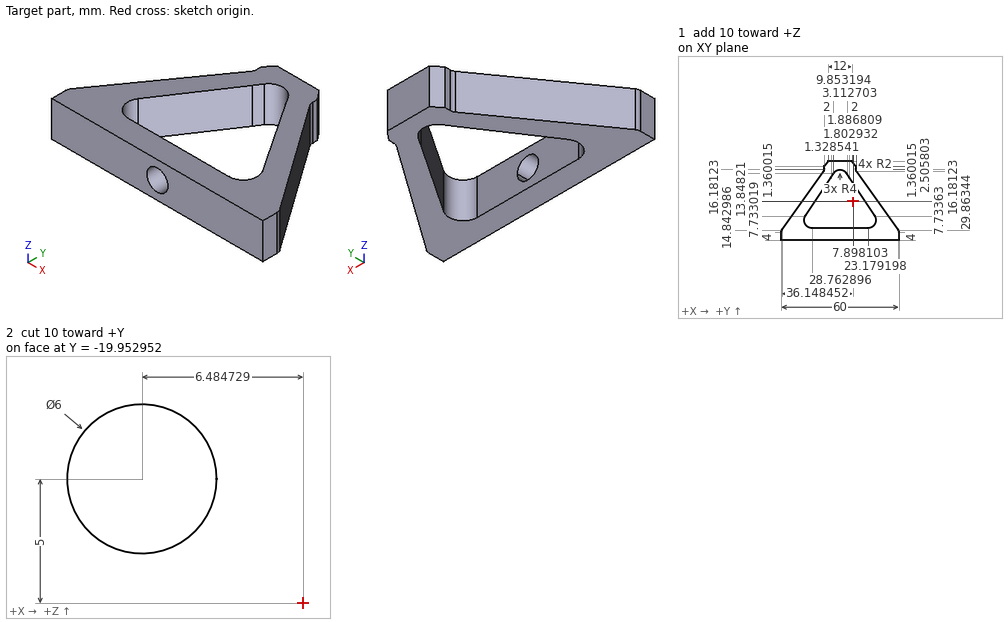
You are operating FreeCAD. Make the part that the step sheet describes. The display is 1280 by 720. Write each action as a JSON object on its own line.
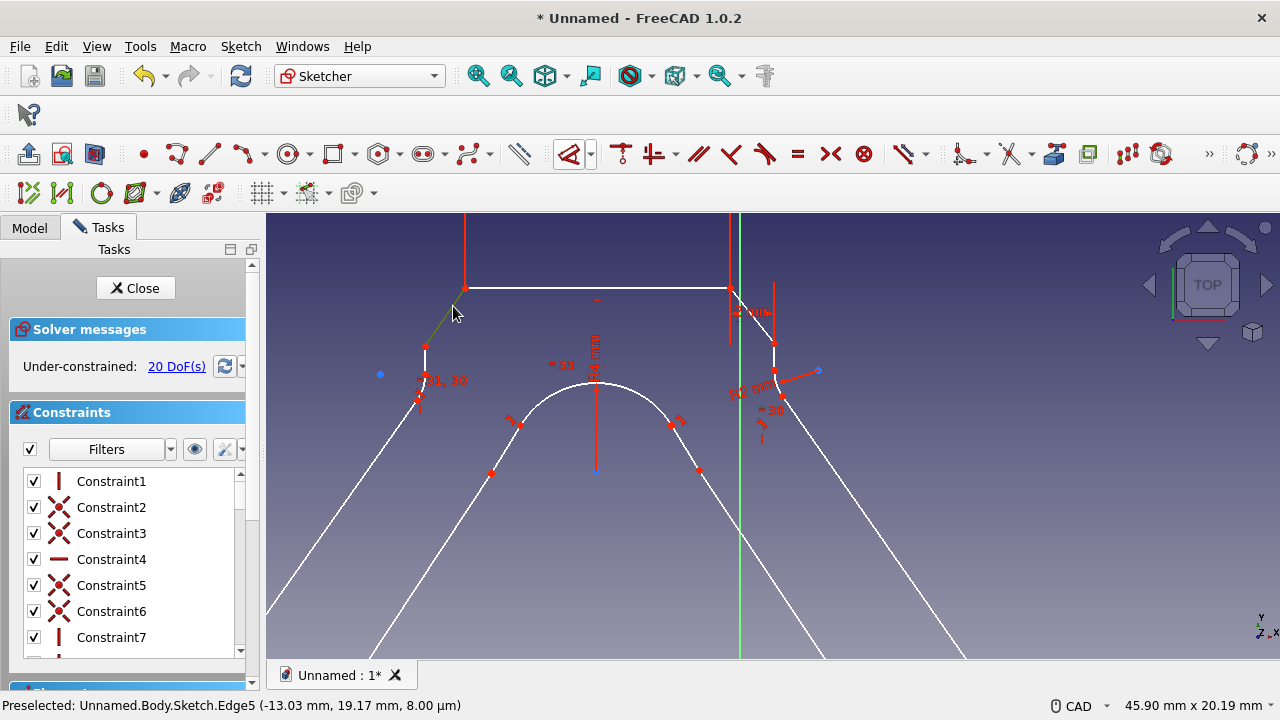
{"action": "key", "text": "l"}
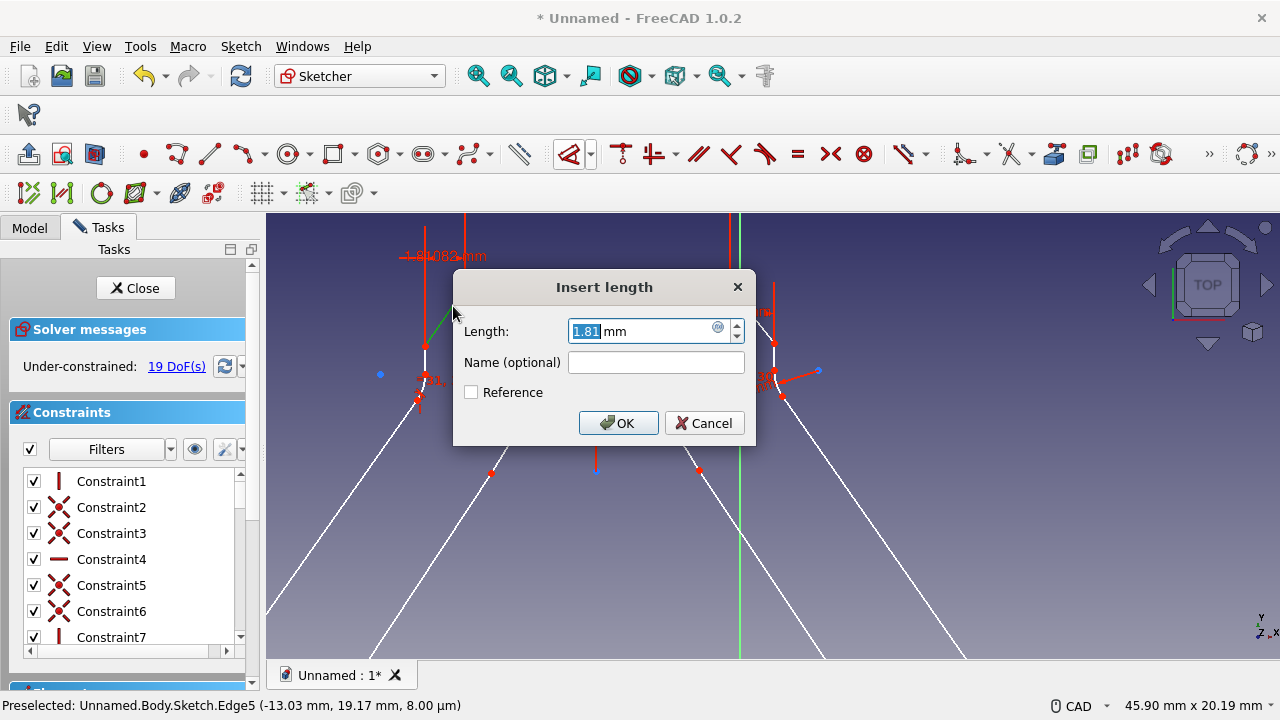
{"action": "type", "text": "2"}
{"action": "key", "text": "Return"}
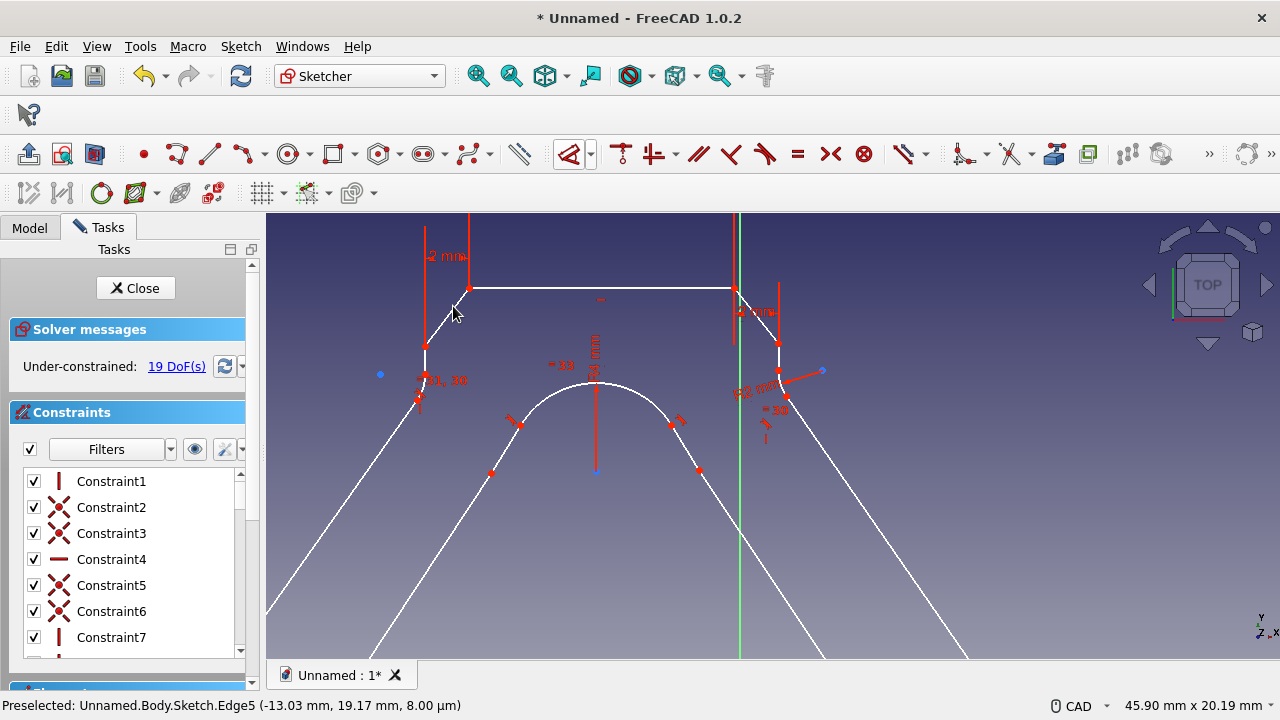
{"action": "scroll", "coordinate": [779, 360], "scroll_direction": "up", "scroll_amount": 2}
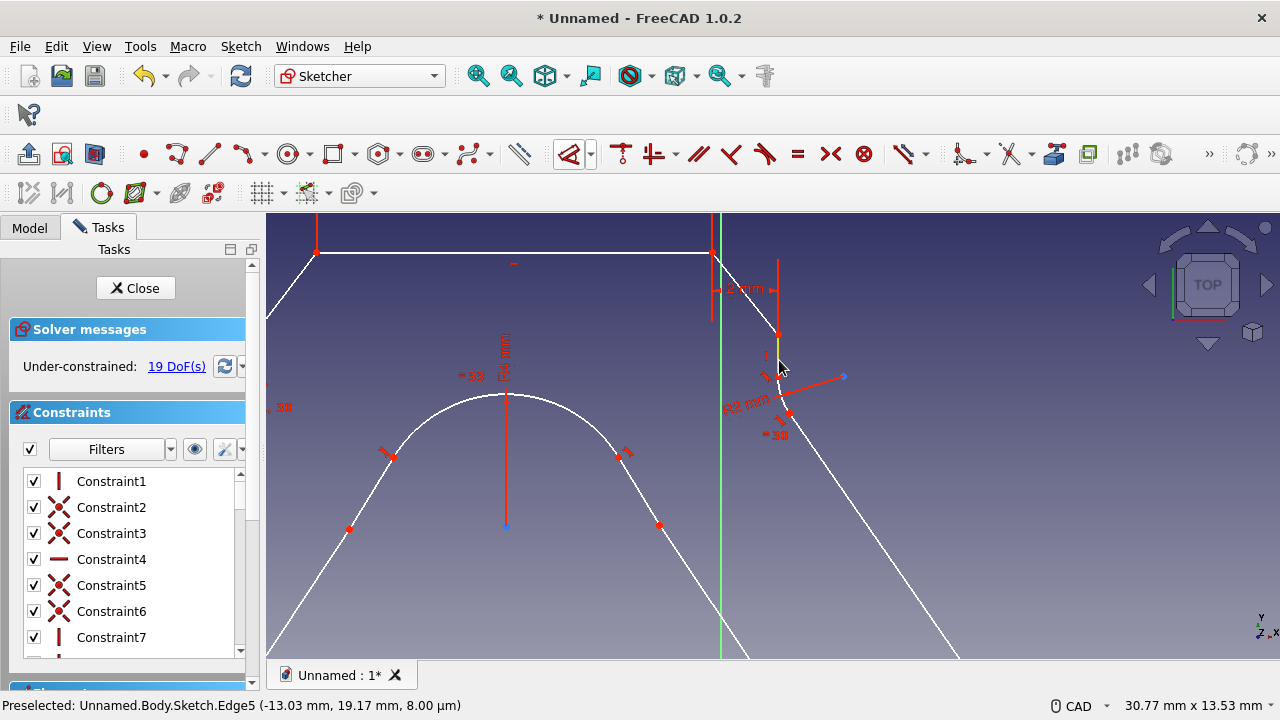
{"action": "left_click", "coordinate": [778, 360]}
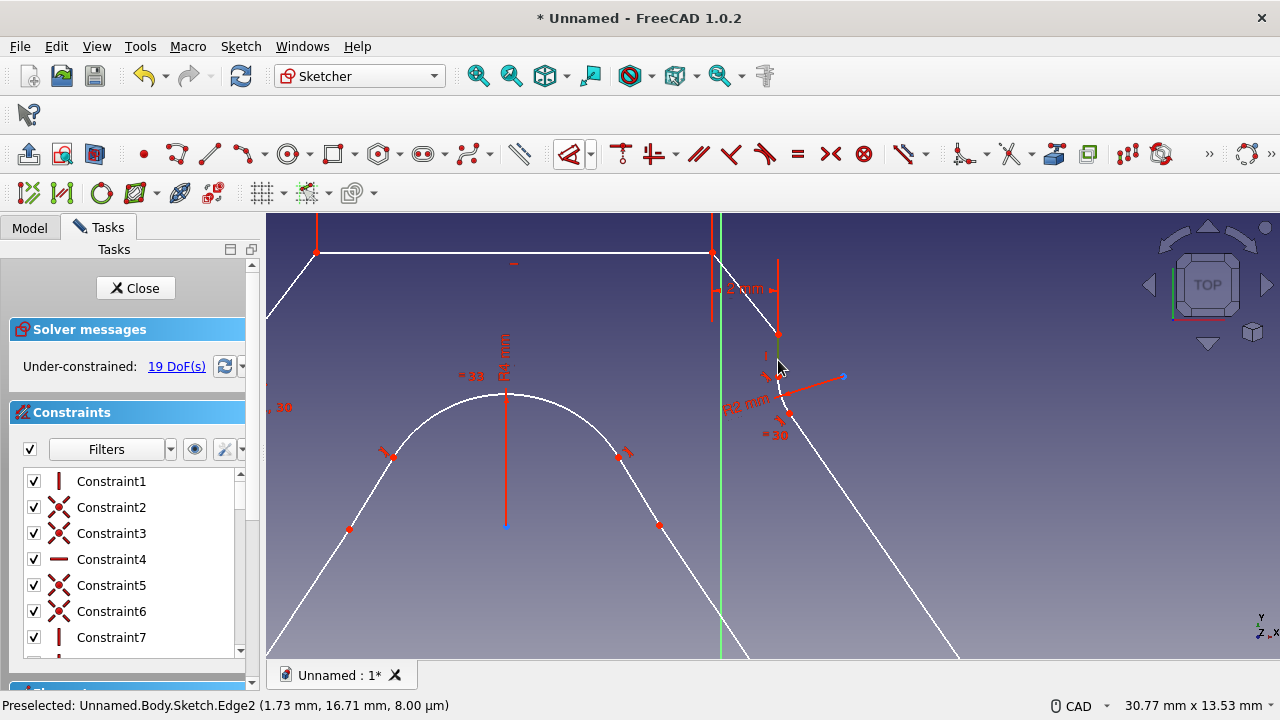
{"action": "key", "text": "i"}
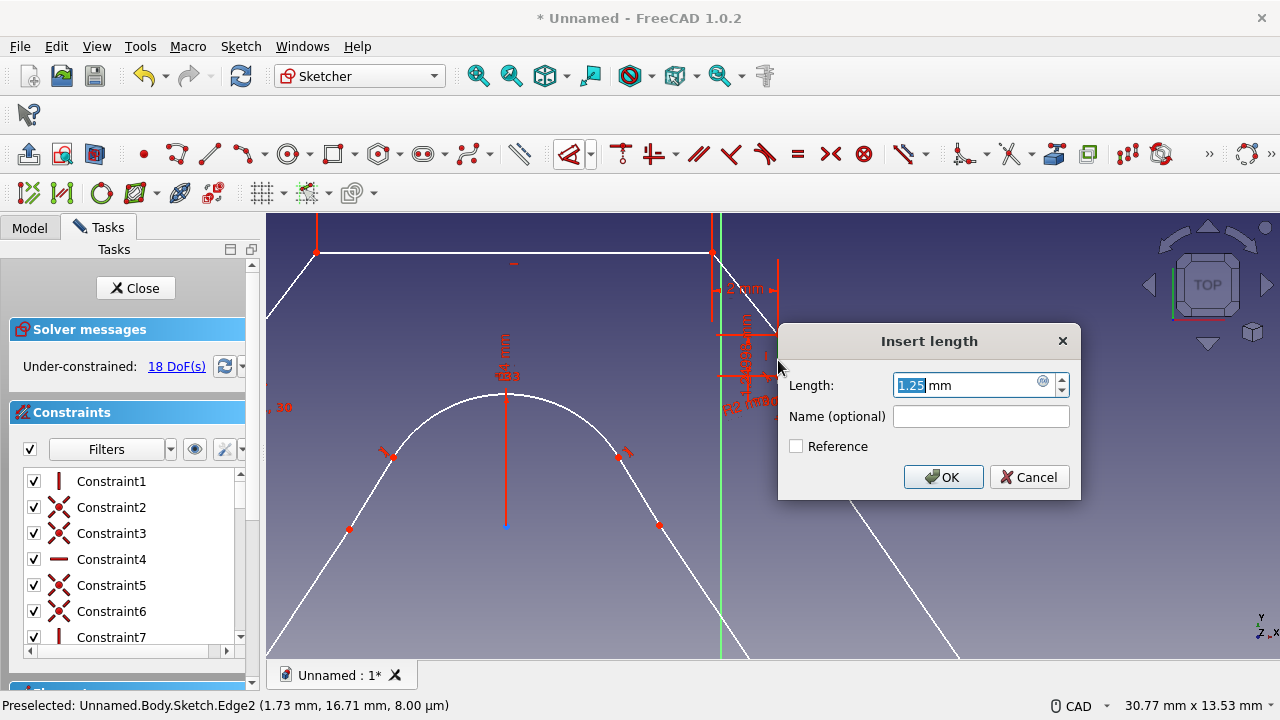
{"action": "type", "text": "1.360015"}
{"action": "key", "text": "Return"}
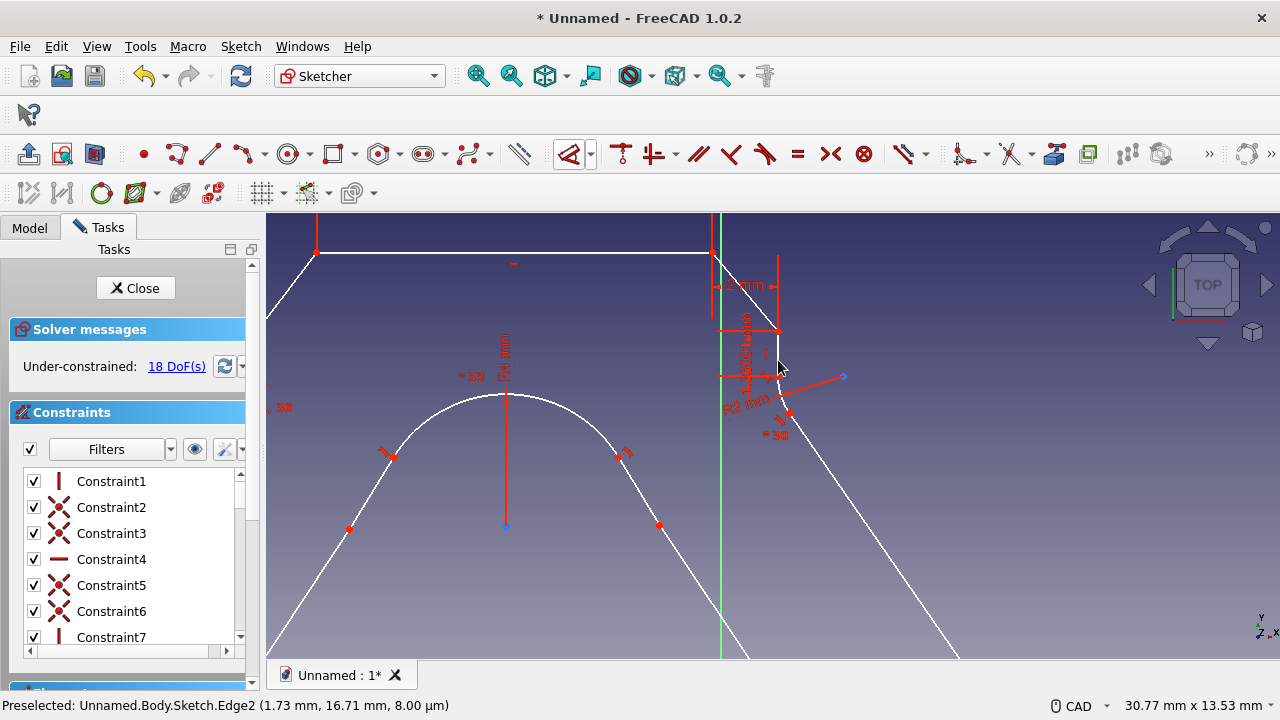
{"action": "scroll", "coordinate": [754, 316], "scroll_direction": "down", "scroll_amount": 8}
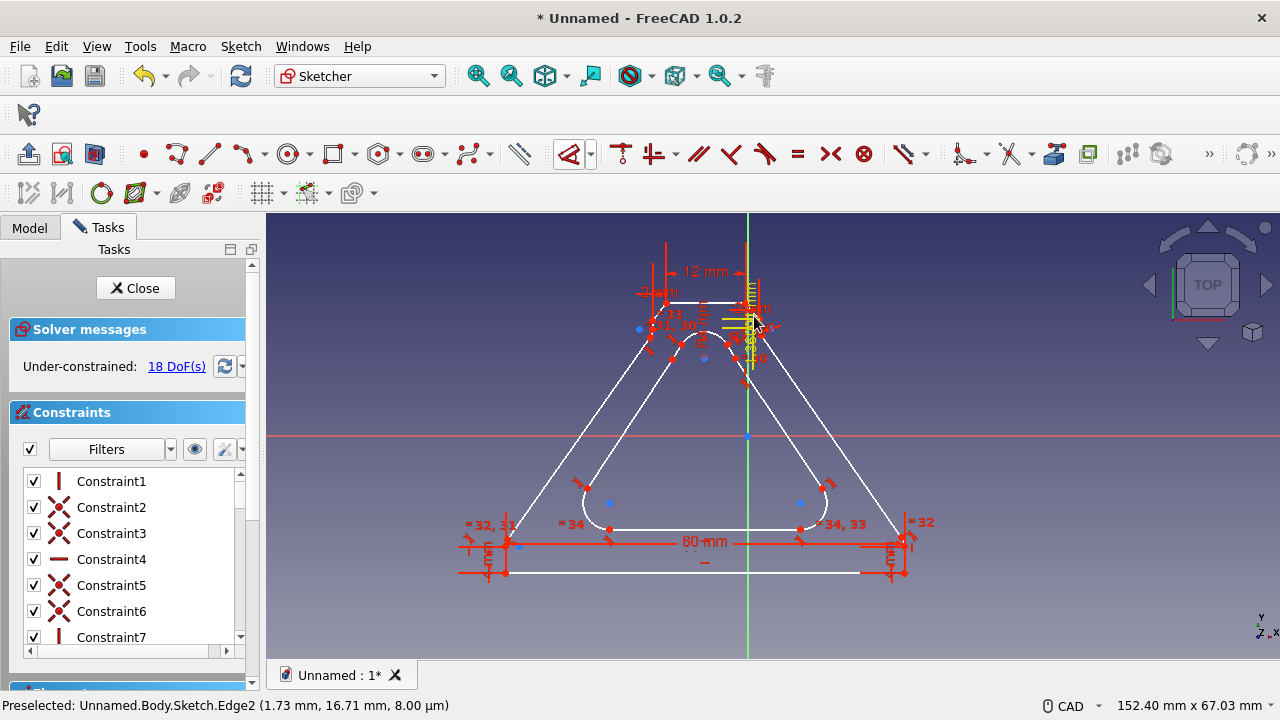
{"action": "scroll", "coordinate": [653, 323], "scroll_direction": "up", "scroll_amount": 9}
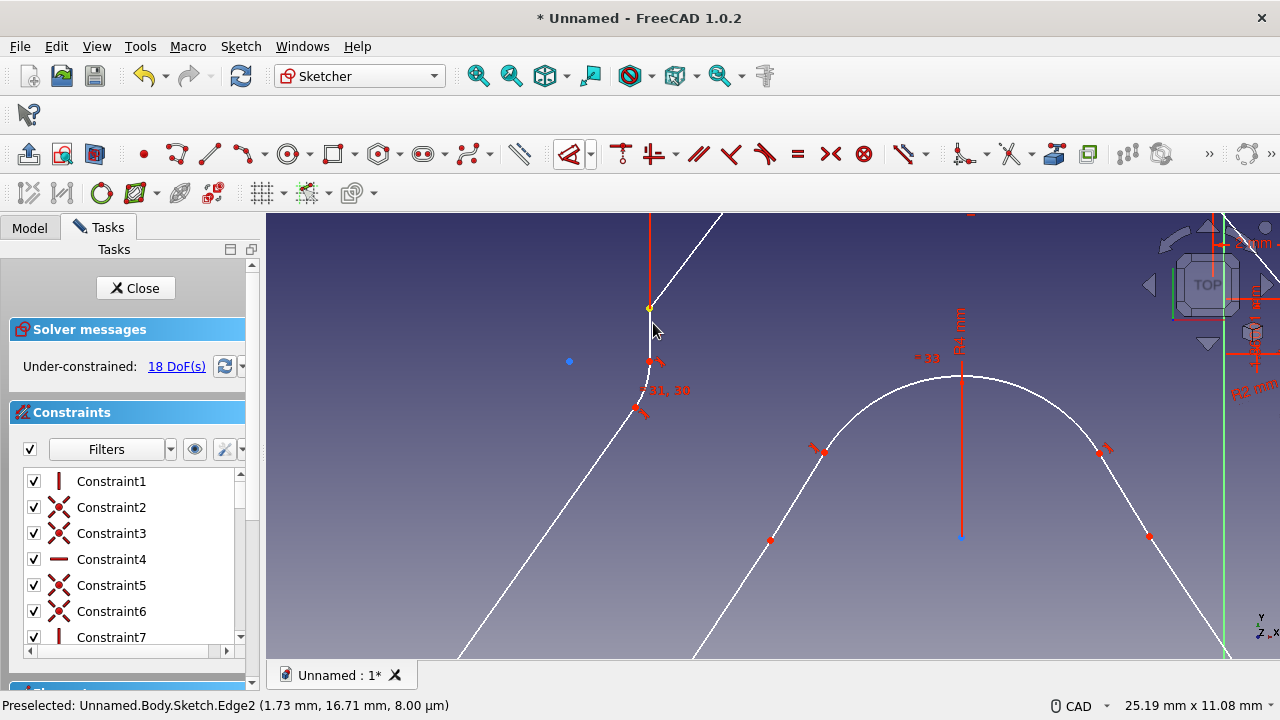
{"action": "left_click", "coordinate": [650, 325]}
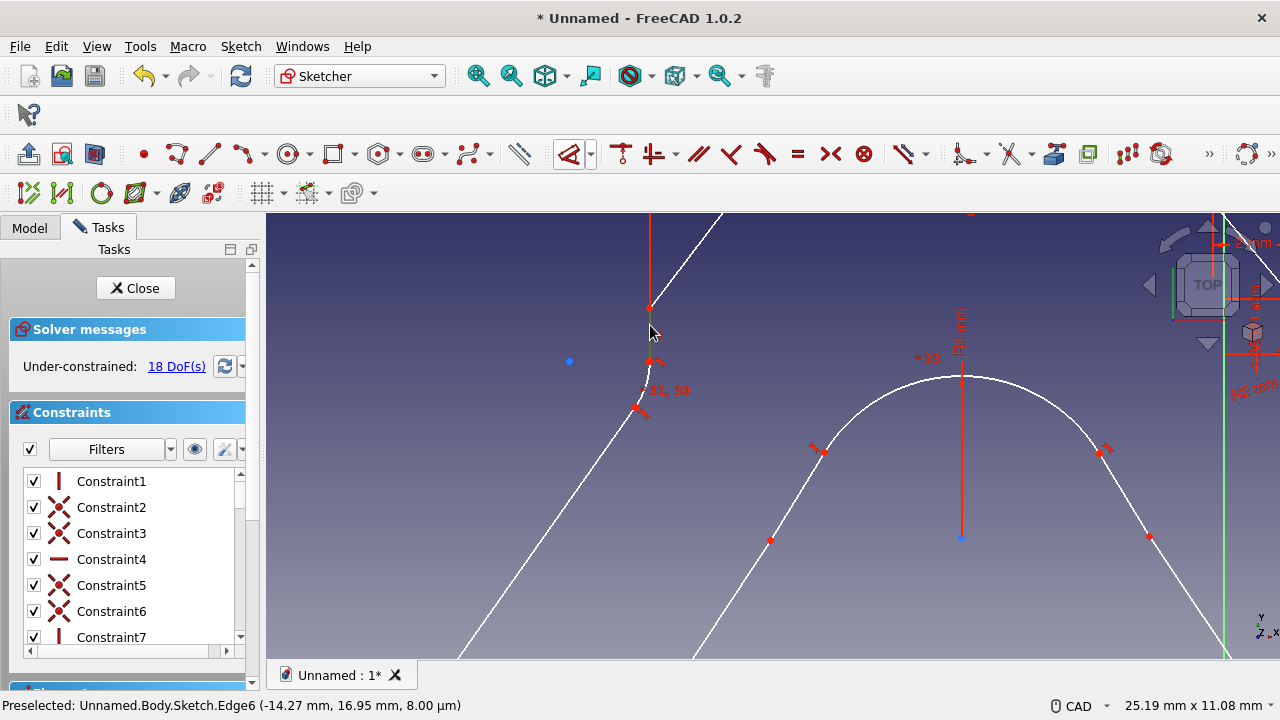
{"action": "left_click", "coordinate": [590, 154]}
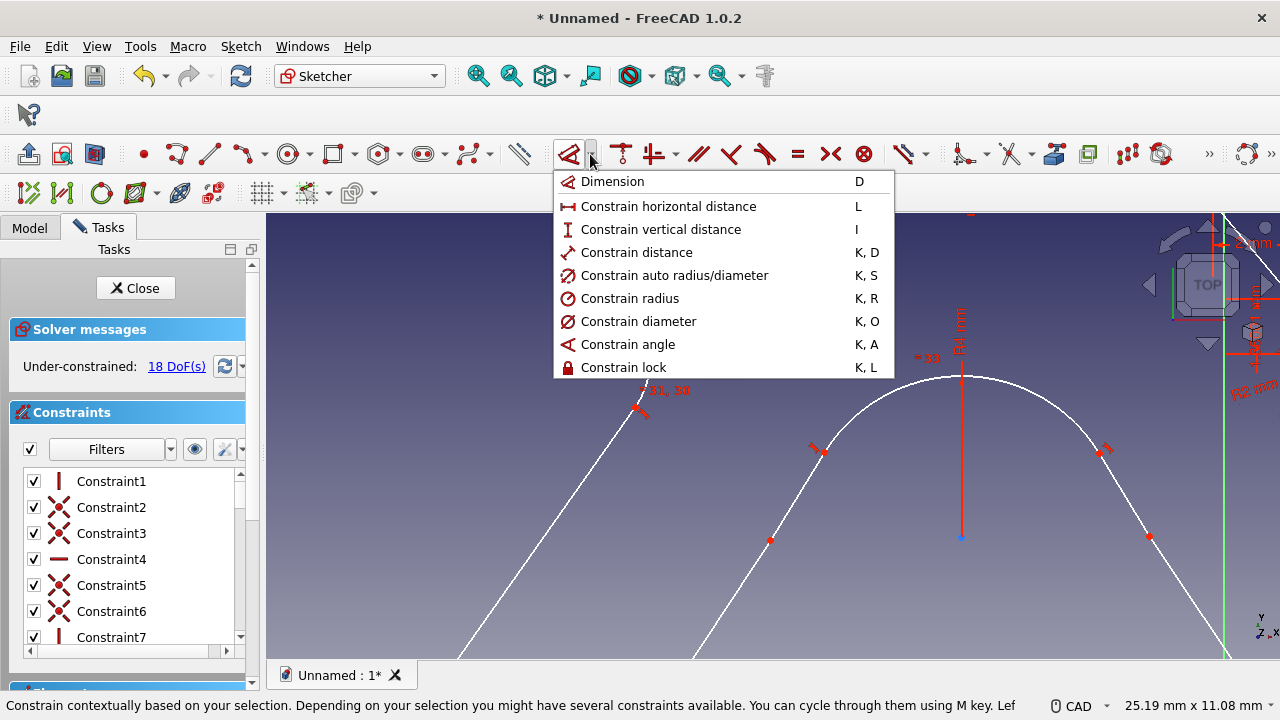
{"action": "left_click", "coordinate": [724, 230]}